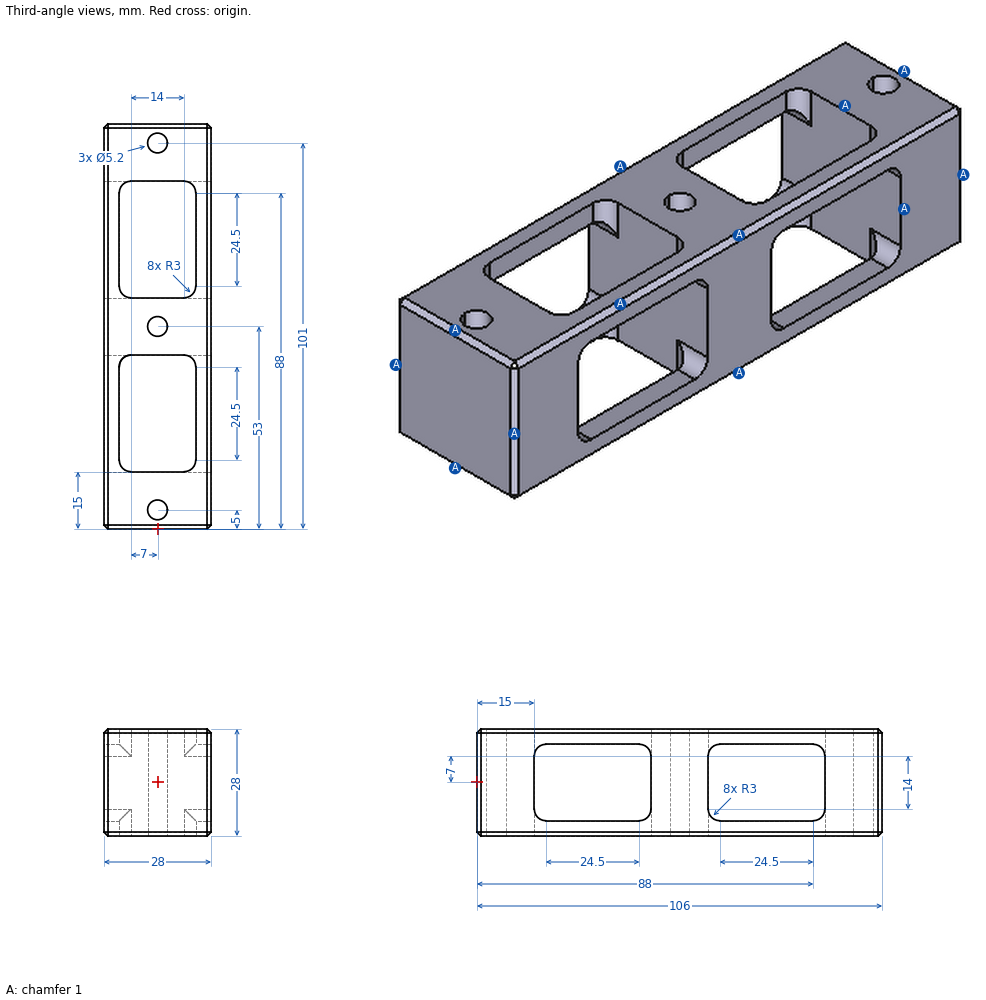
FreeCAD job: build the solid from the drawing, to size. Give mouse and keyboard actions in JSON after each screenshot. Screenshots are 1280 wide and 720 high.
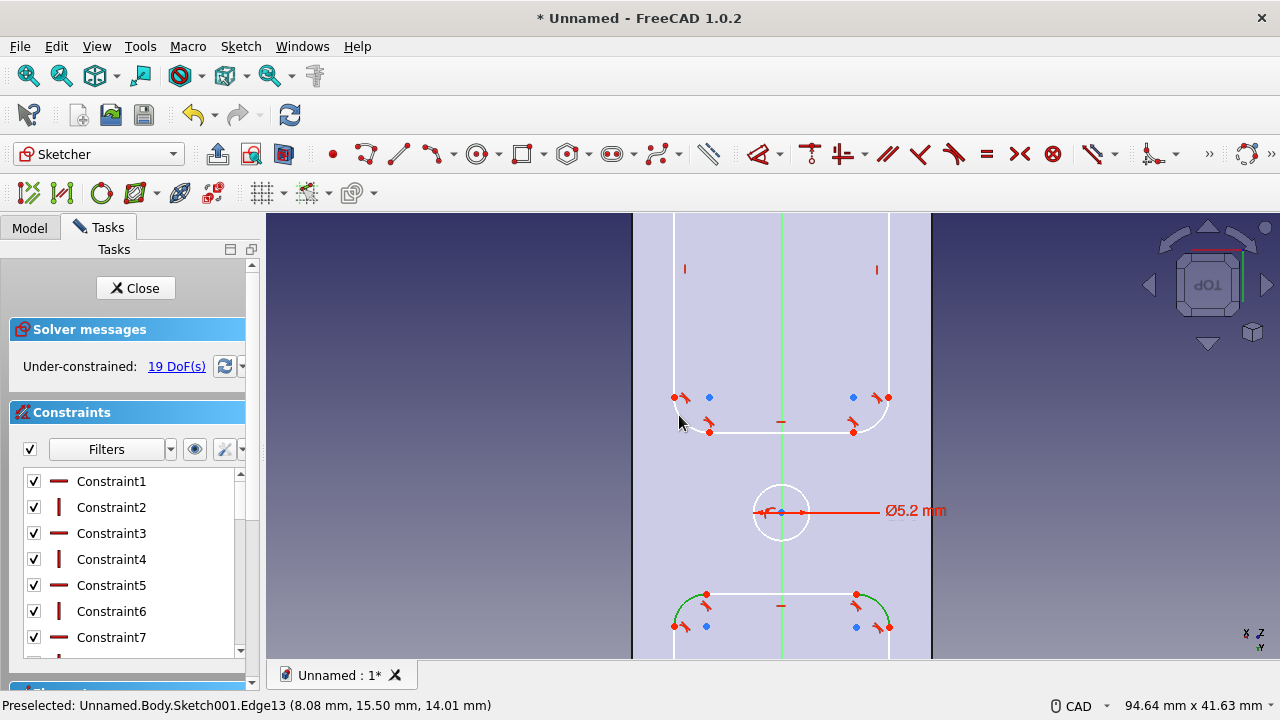
{"action": "left_click", "coordinate": [678, 413]}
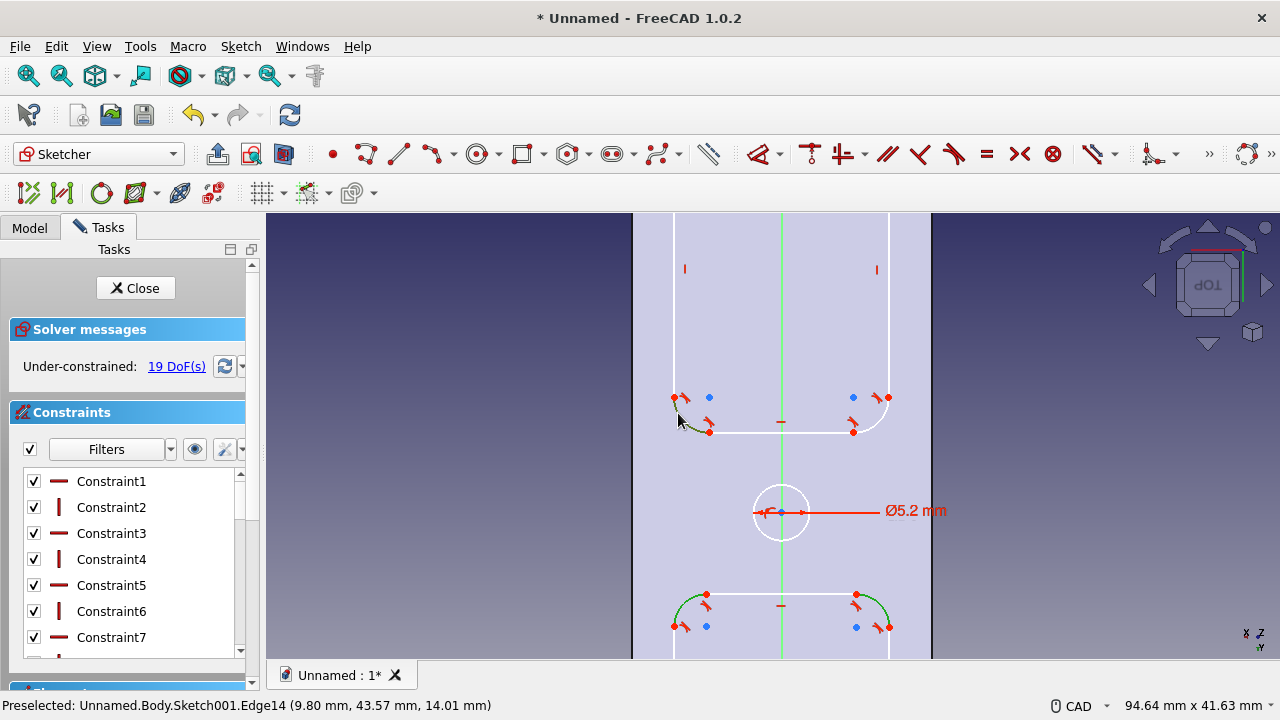
{"action": "left_click", "coordinate": [870, 429]}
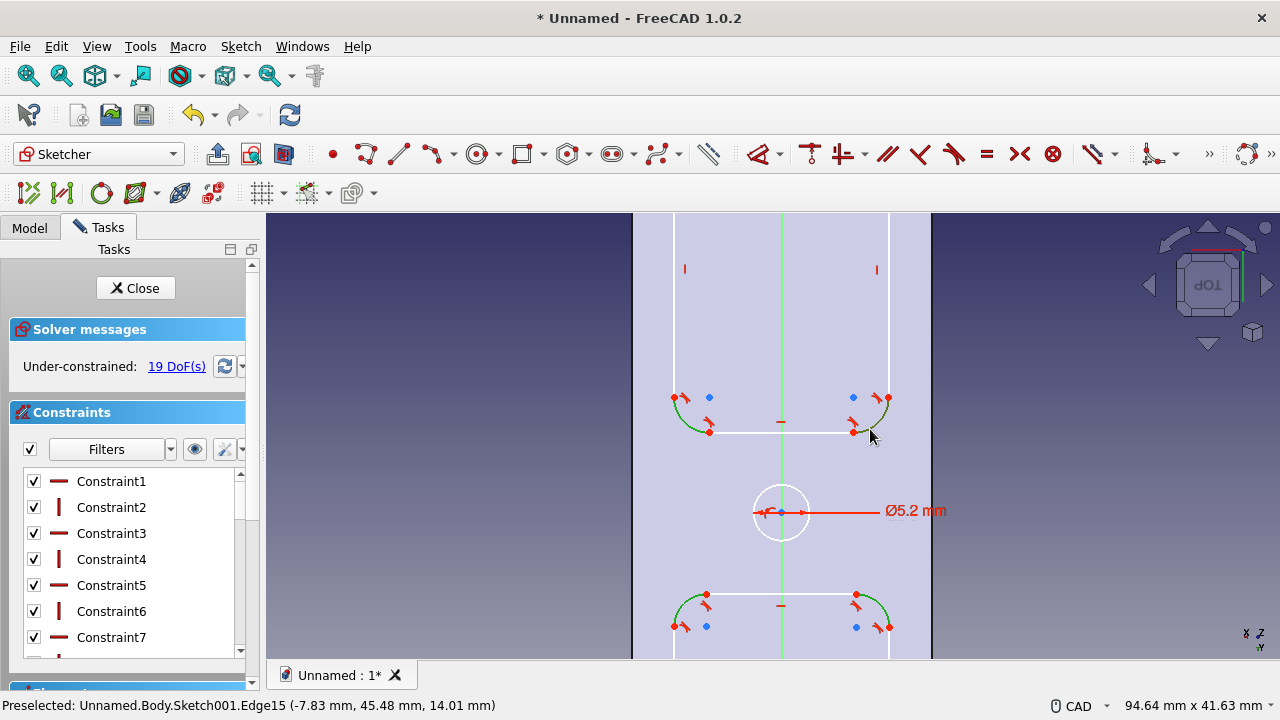
{"action": "scroll", "coordinate": [679, 416], "scroll_direction": "down", "scroll_amount": 7}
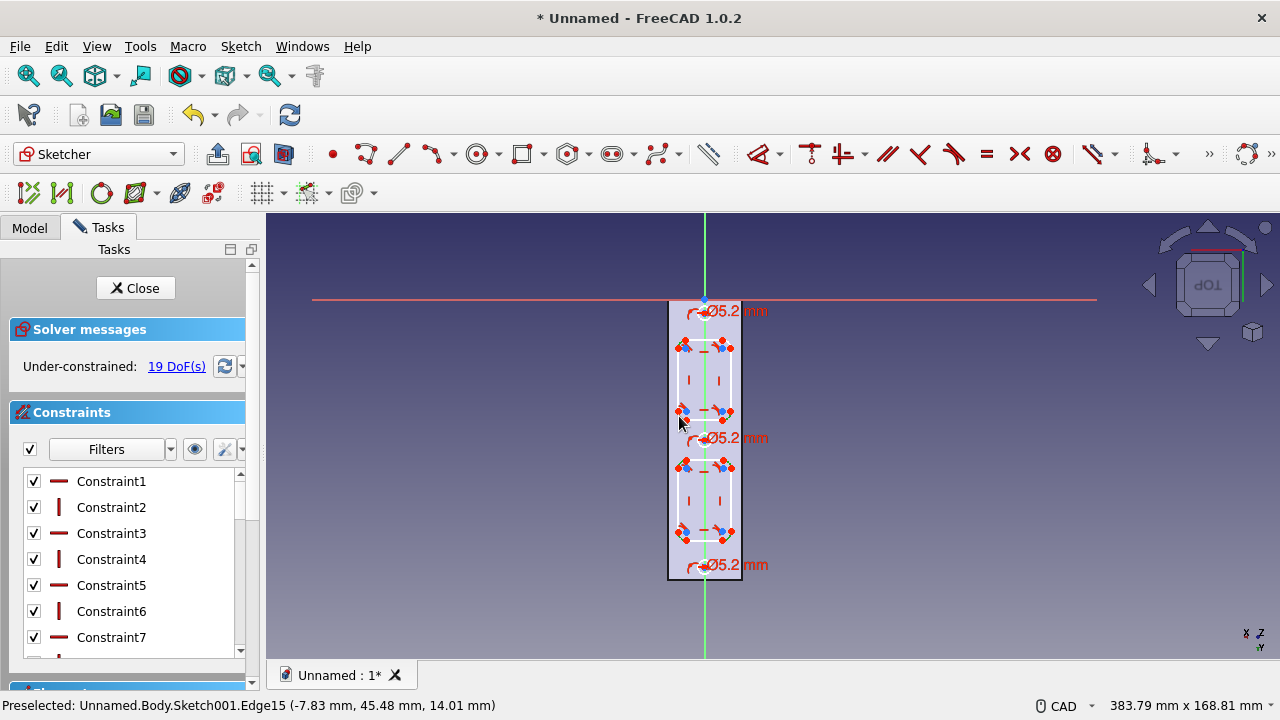
{"action": "scroll", "coordinate": [730, 345], "scroll_direction": "up", "scroll_amount": 7}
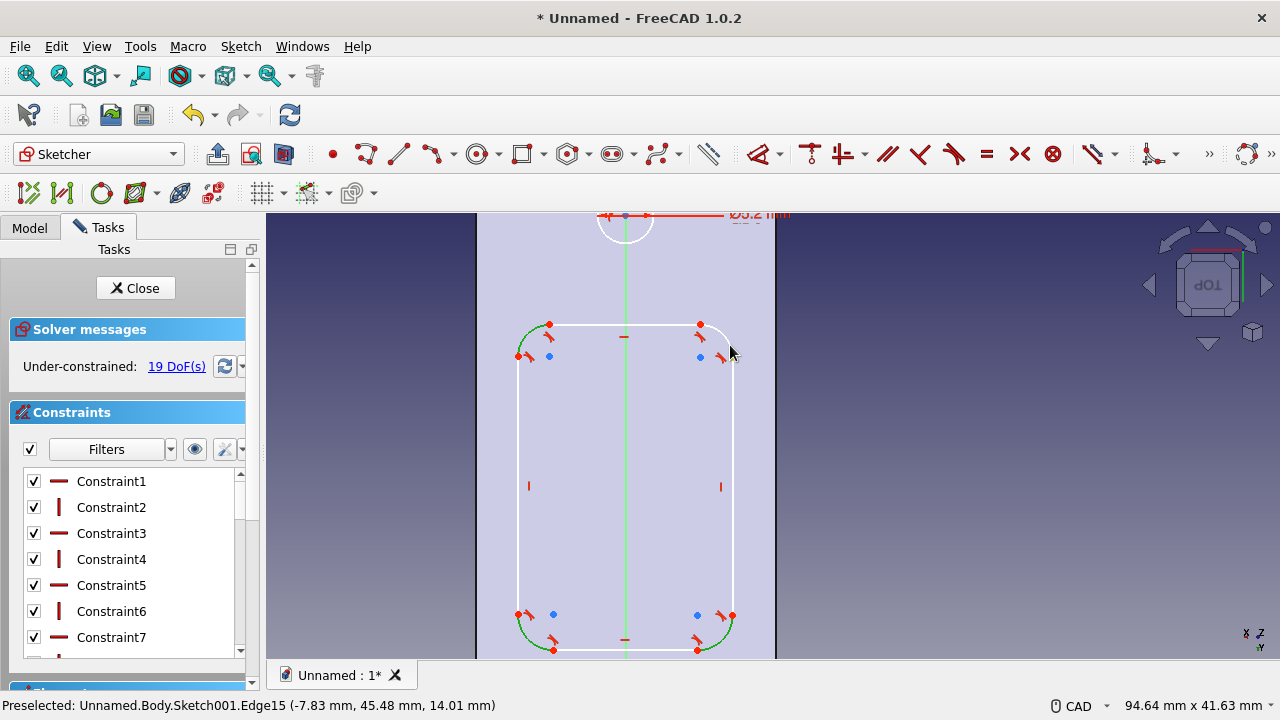
{"action": "left_click", "coordinate": [729, 343]}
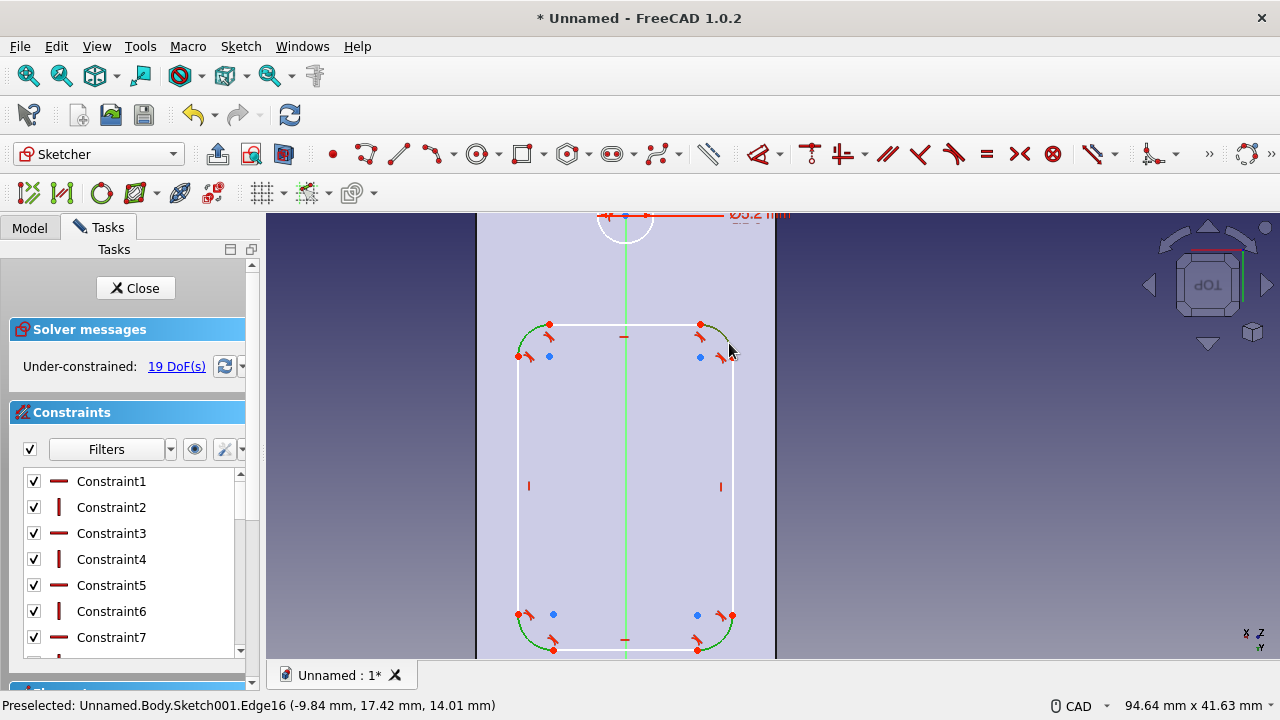
{"action": "key", "text": "e"}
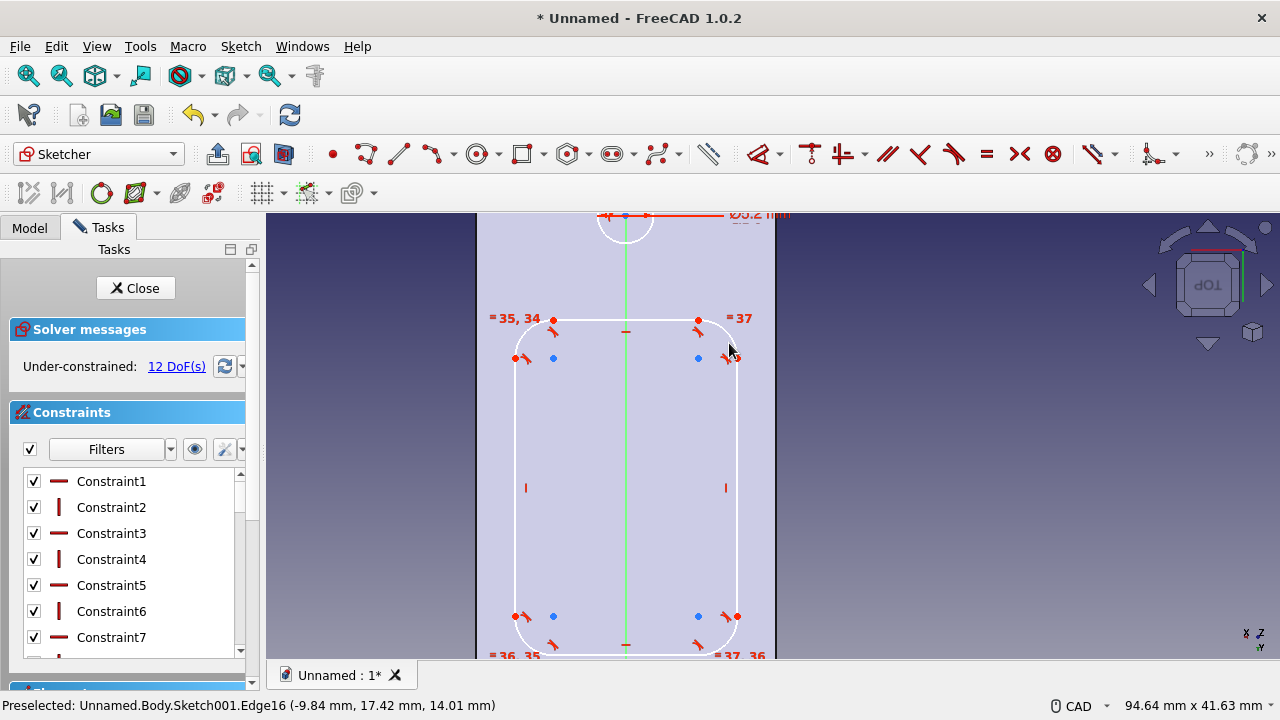
{"action": "key", "text": "d"}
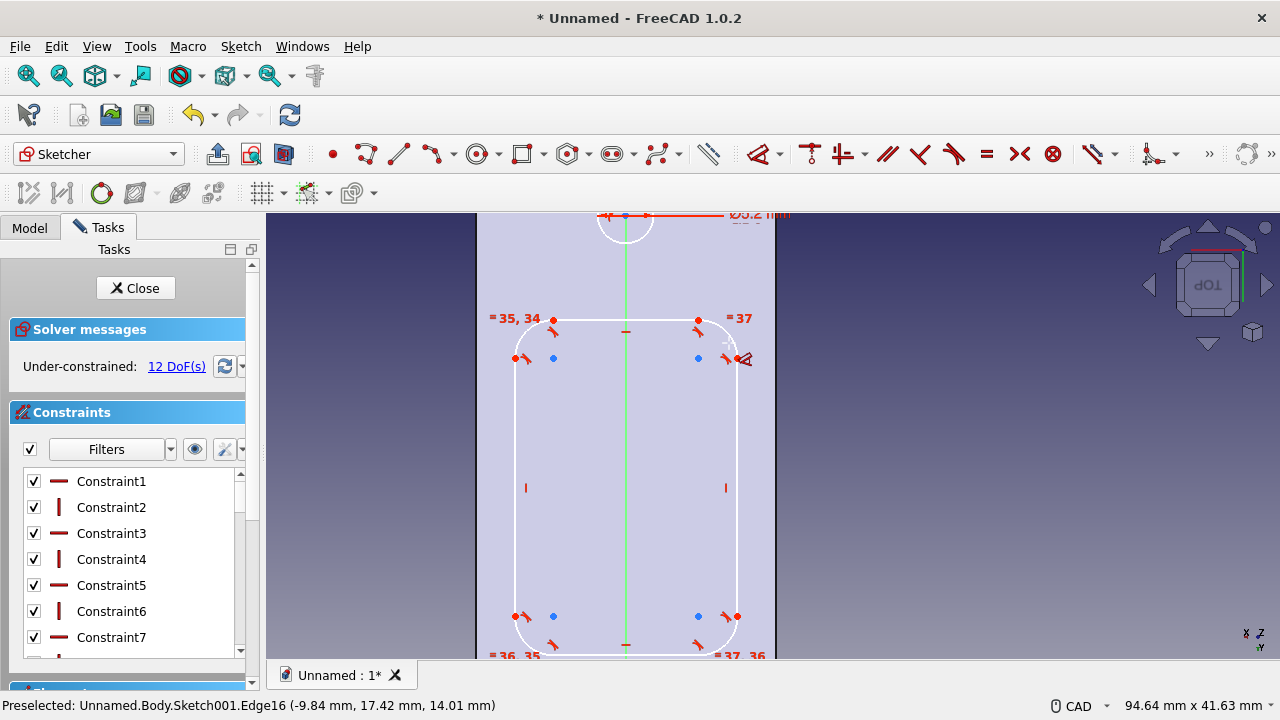
{"action": "scroll", "coordinate": [730, 344], "scroll_direction": "down", "scroll_amount": 7}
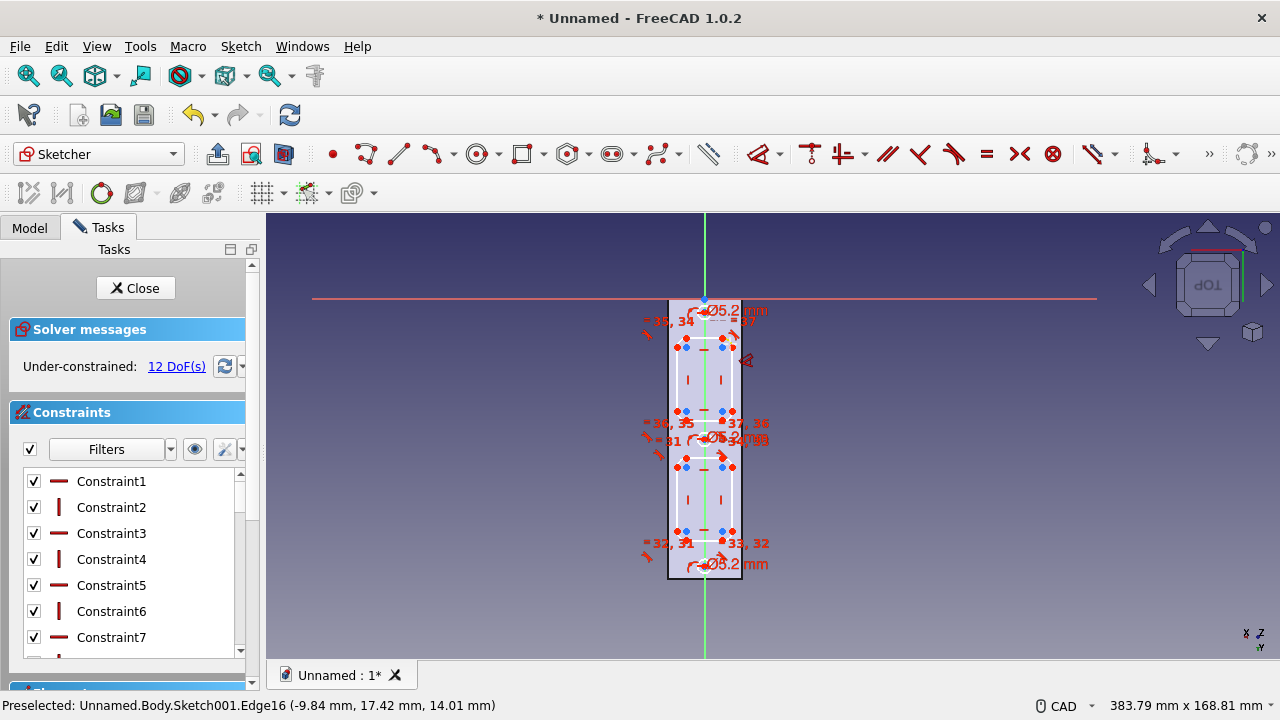
{"action": "scroll", "coordinate": [683, 459], "scroll_direction": "up", "scroll_amount": 9}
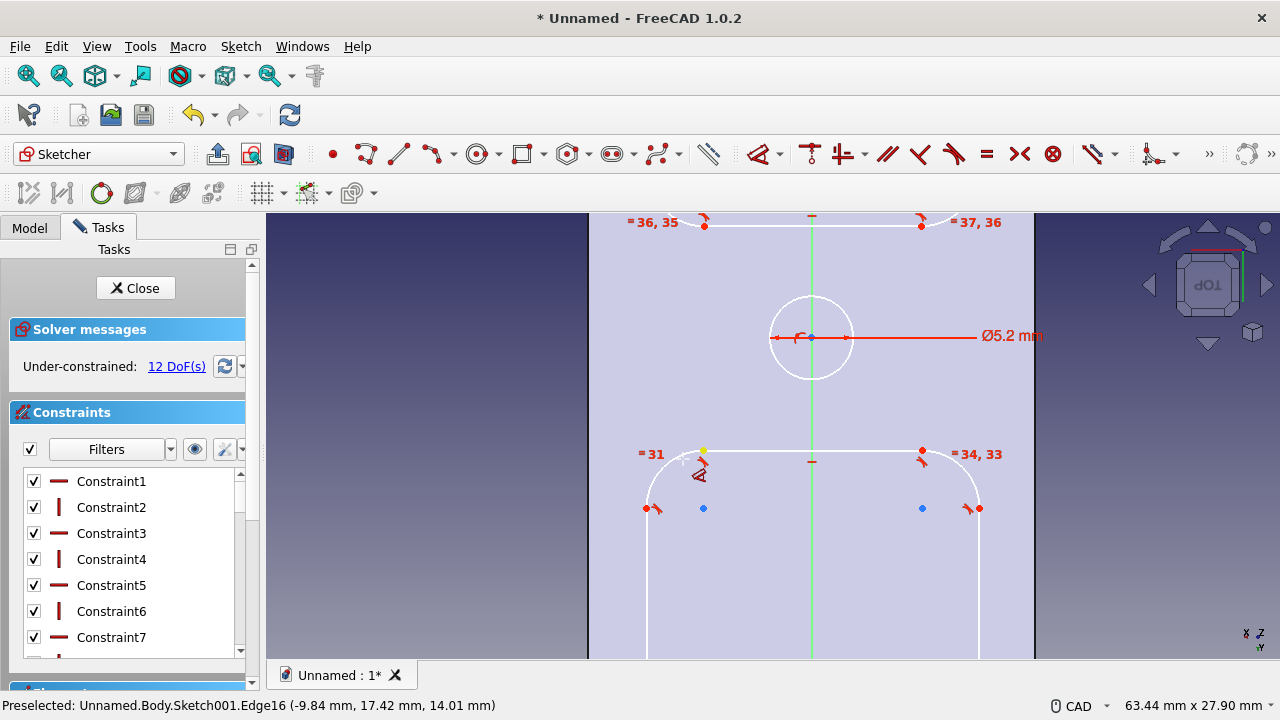
{"action": "left_click", "coordinate": [678, 457]}
{"action": "left_click", "coordinate": [663, 428]}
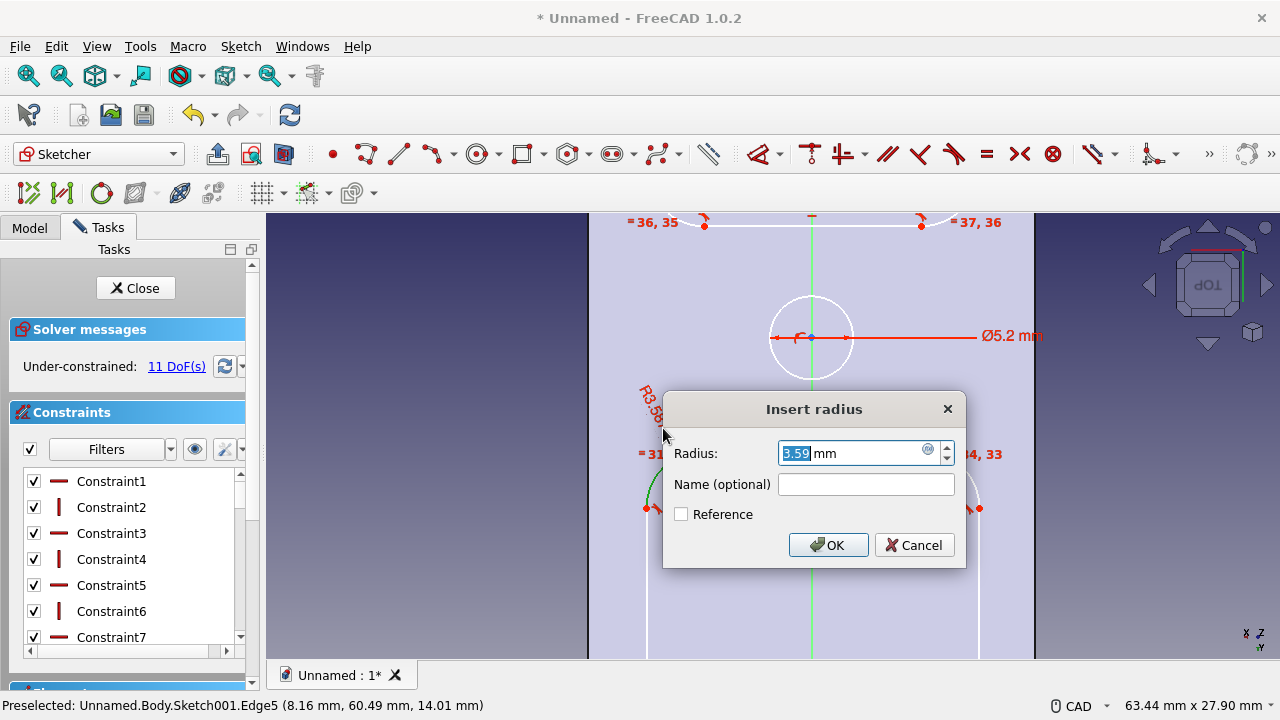
{"action": "type", "text": "3"}
{"action": "key", "text": "Return"}